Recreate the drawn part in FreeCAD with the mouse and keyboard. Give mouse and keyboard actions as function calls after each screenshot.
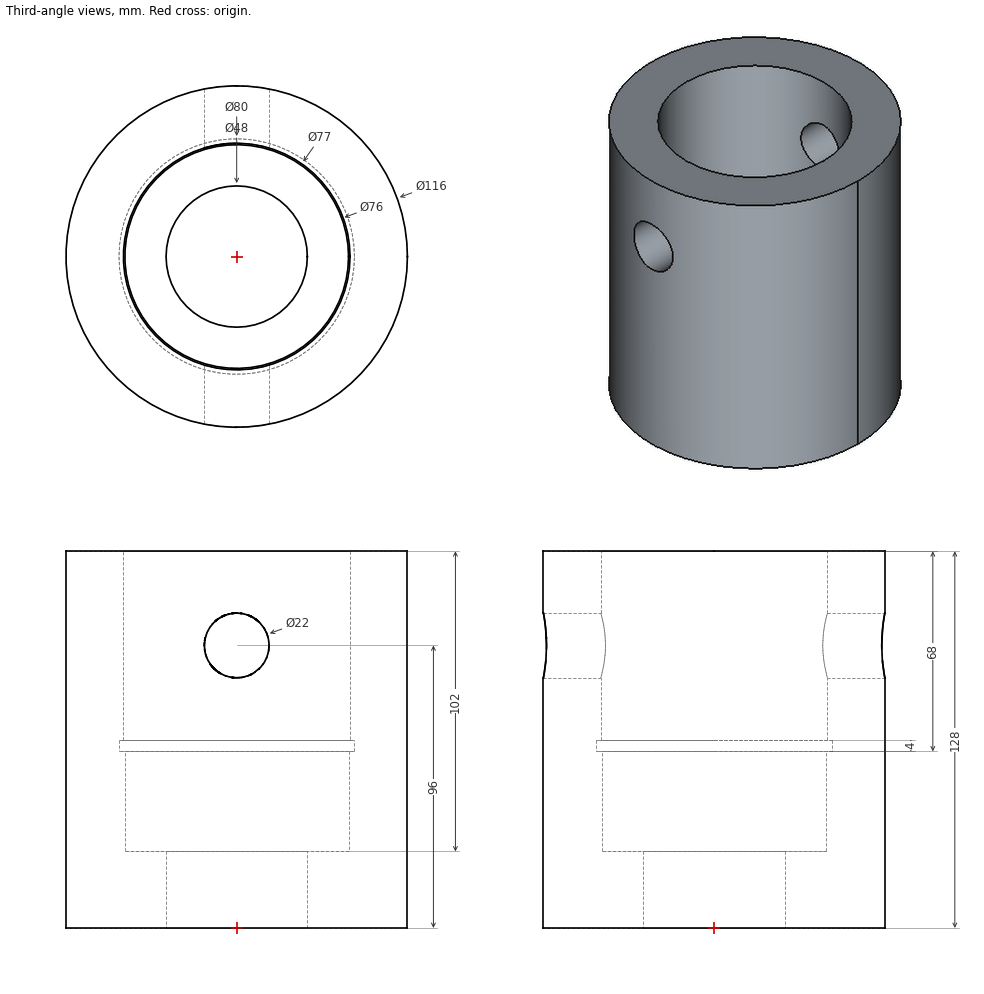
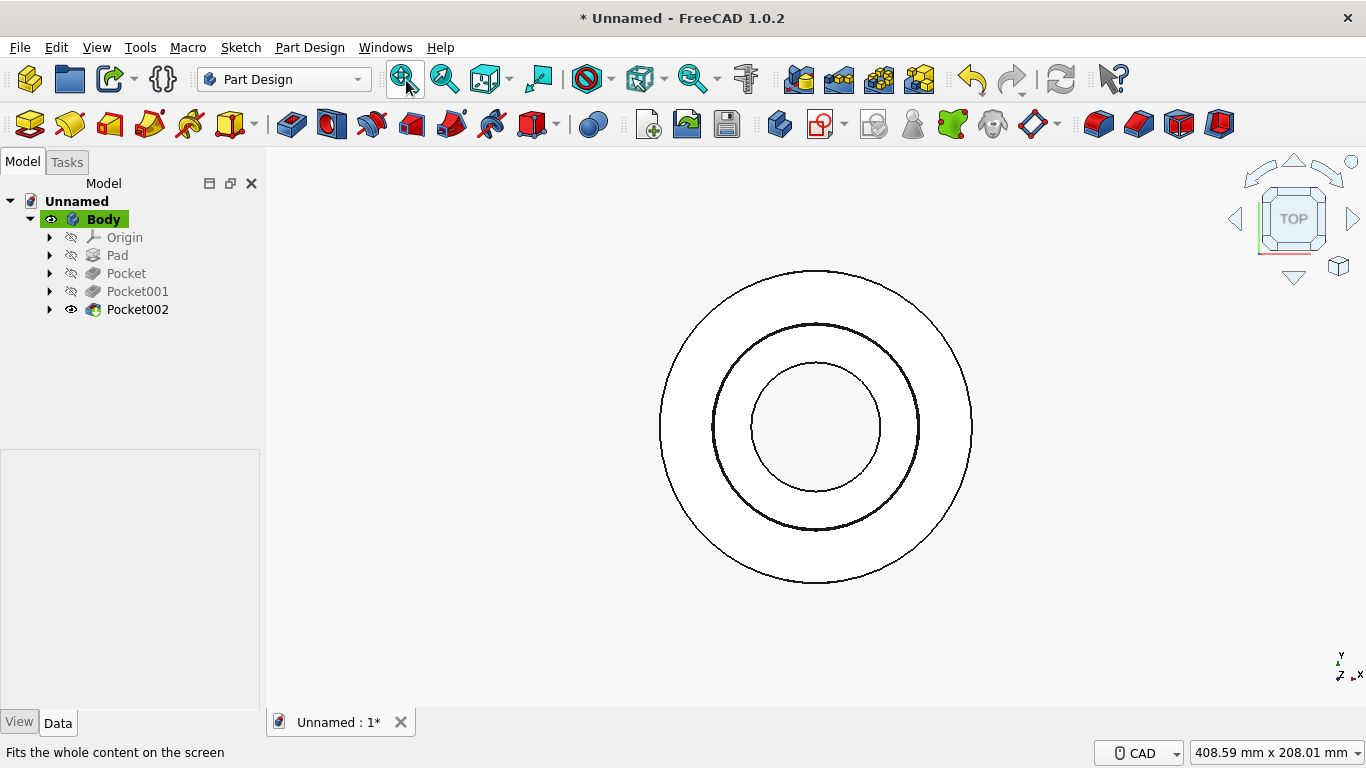
key(1)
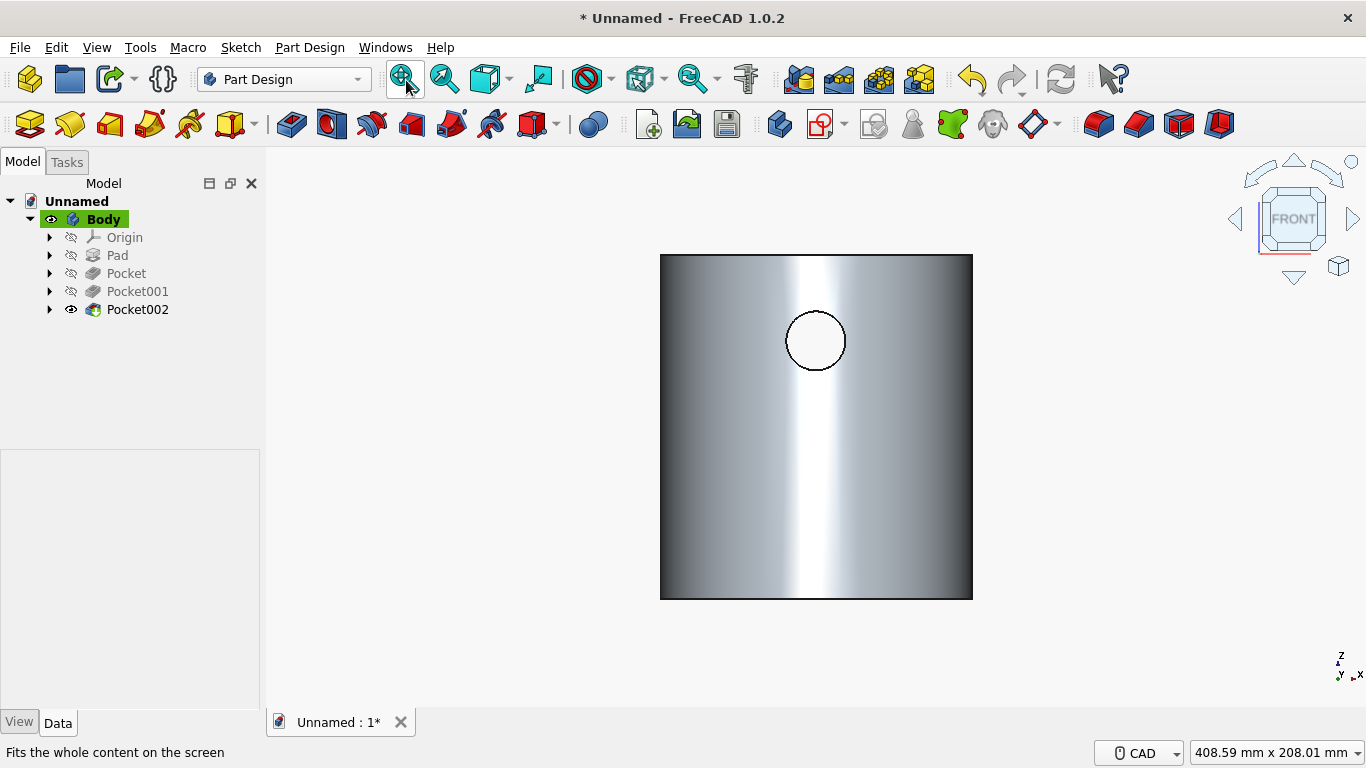
click(50, 237)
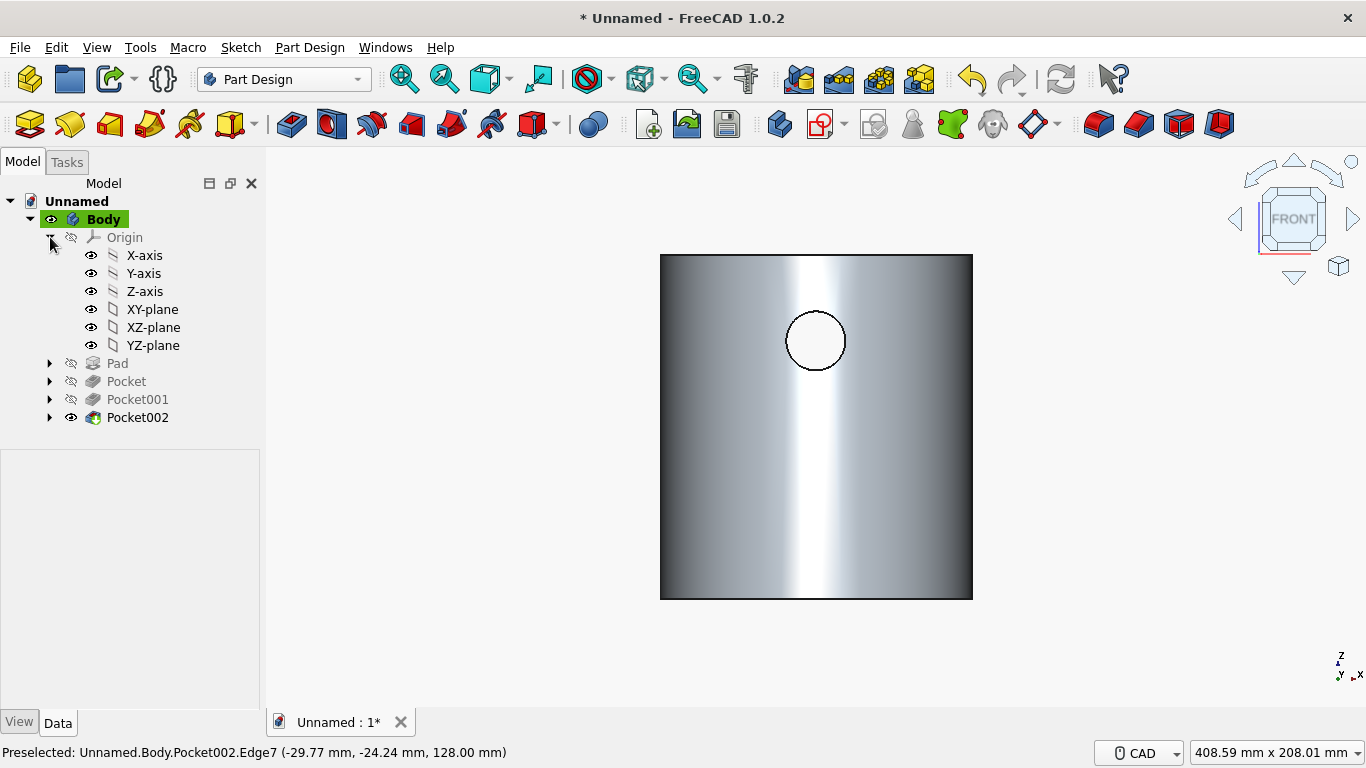
click(136, 309)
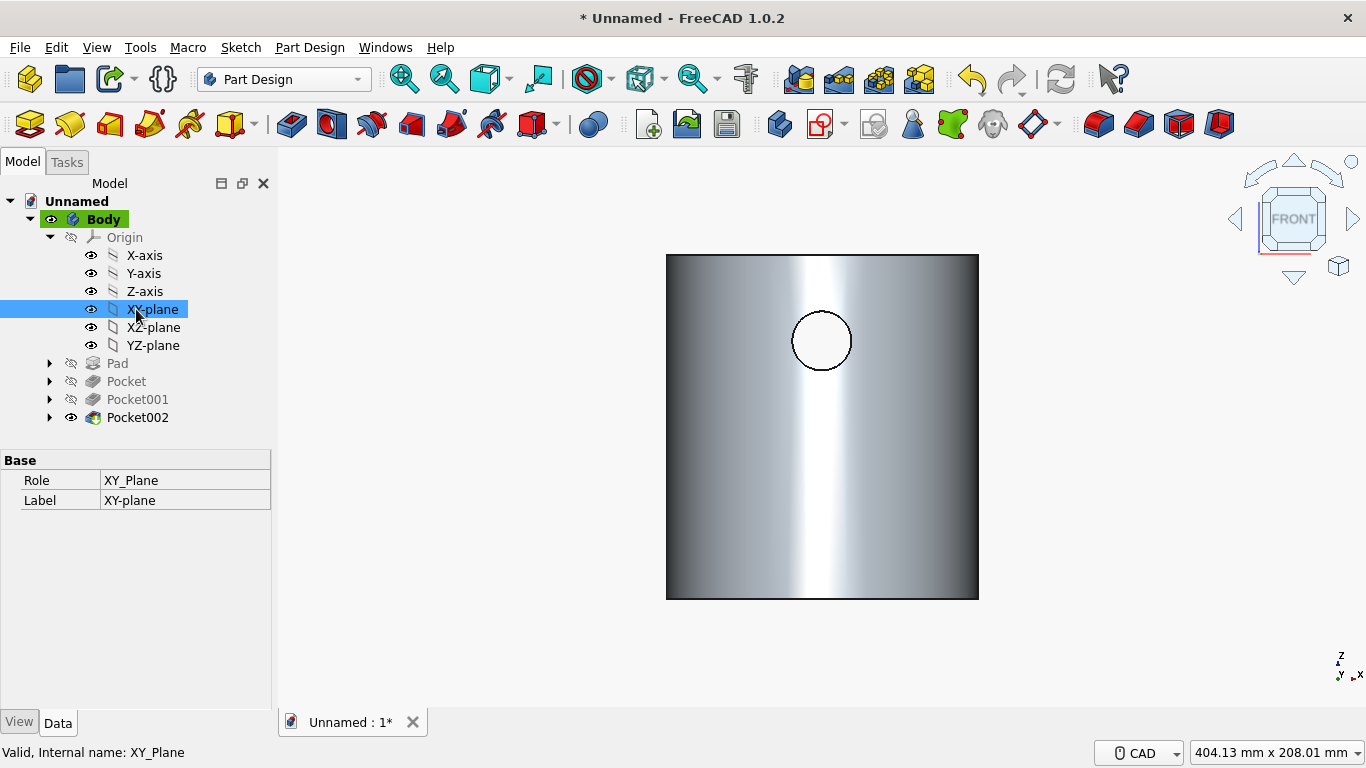
click(1034, 124)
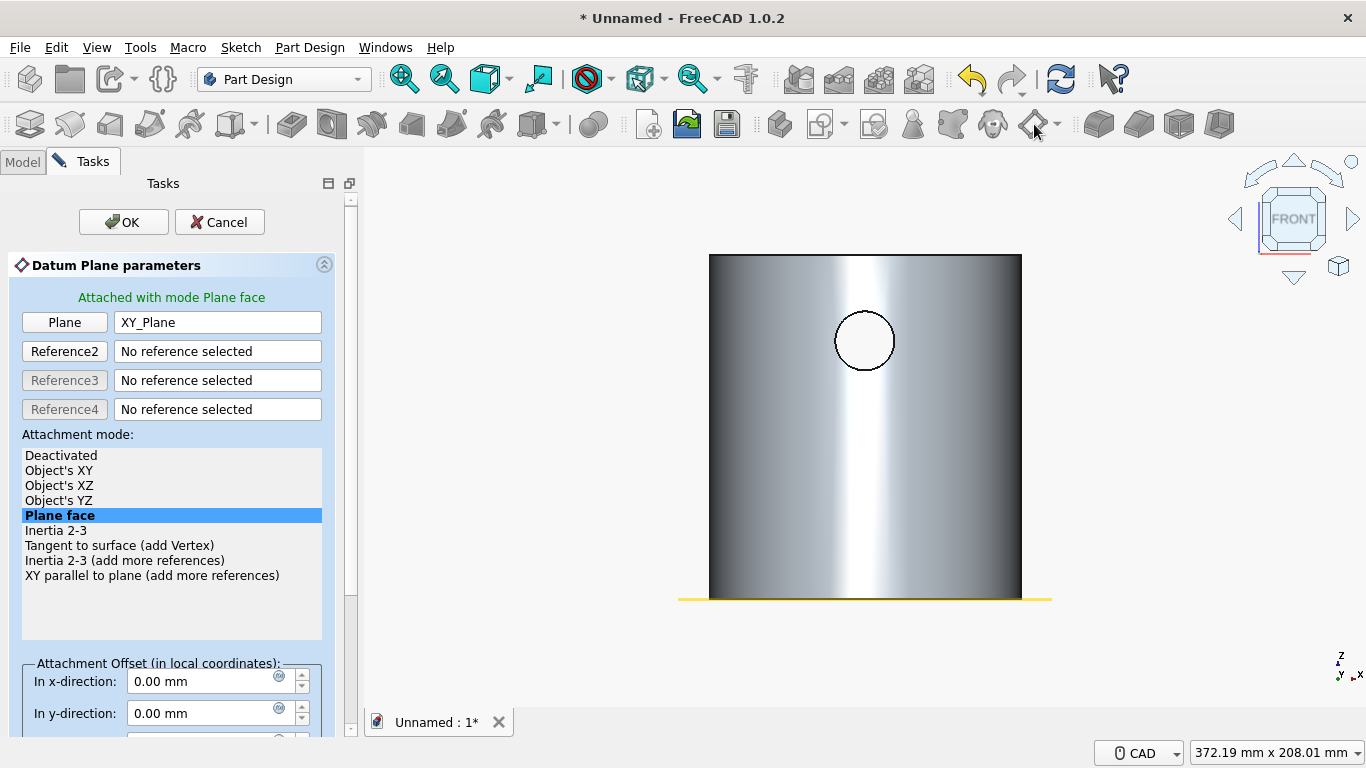
scroll(351, 464, down, 2)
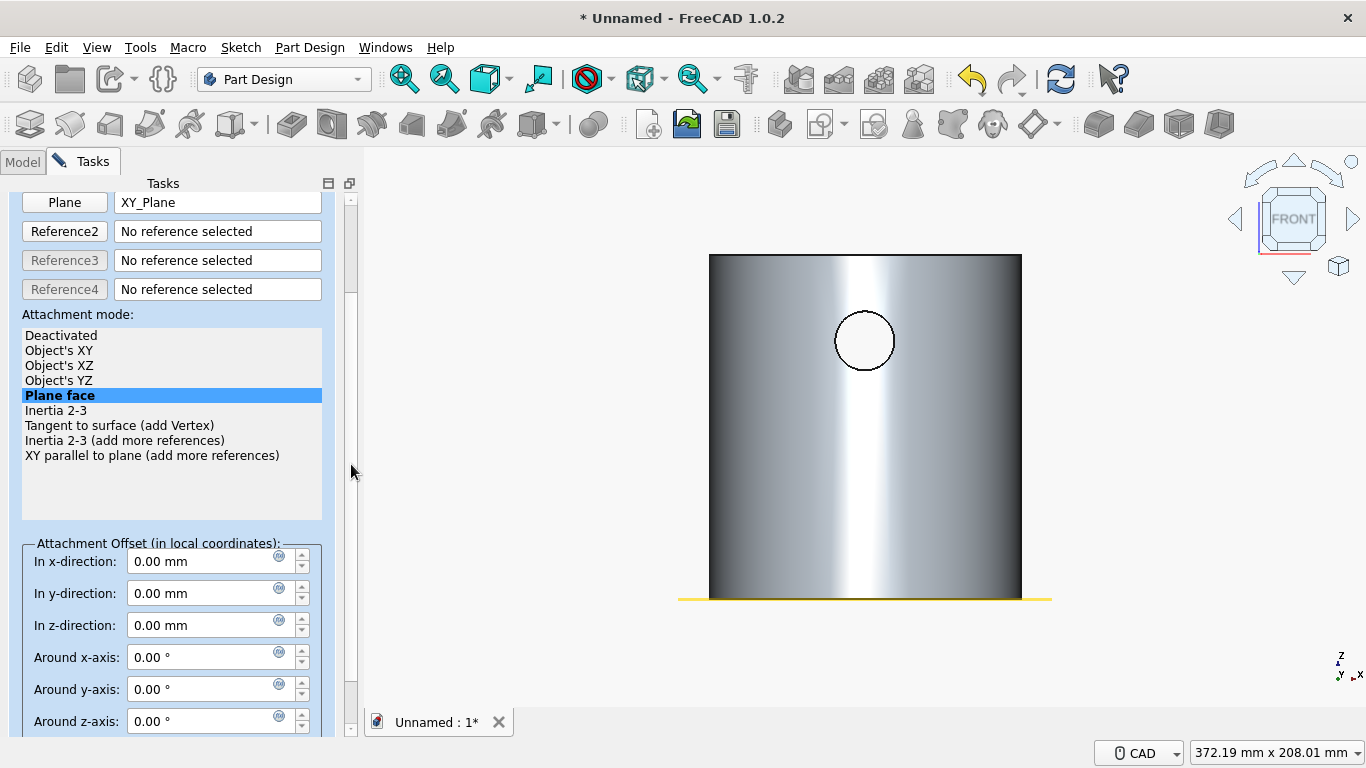
triple_click(210, 625)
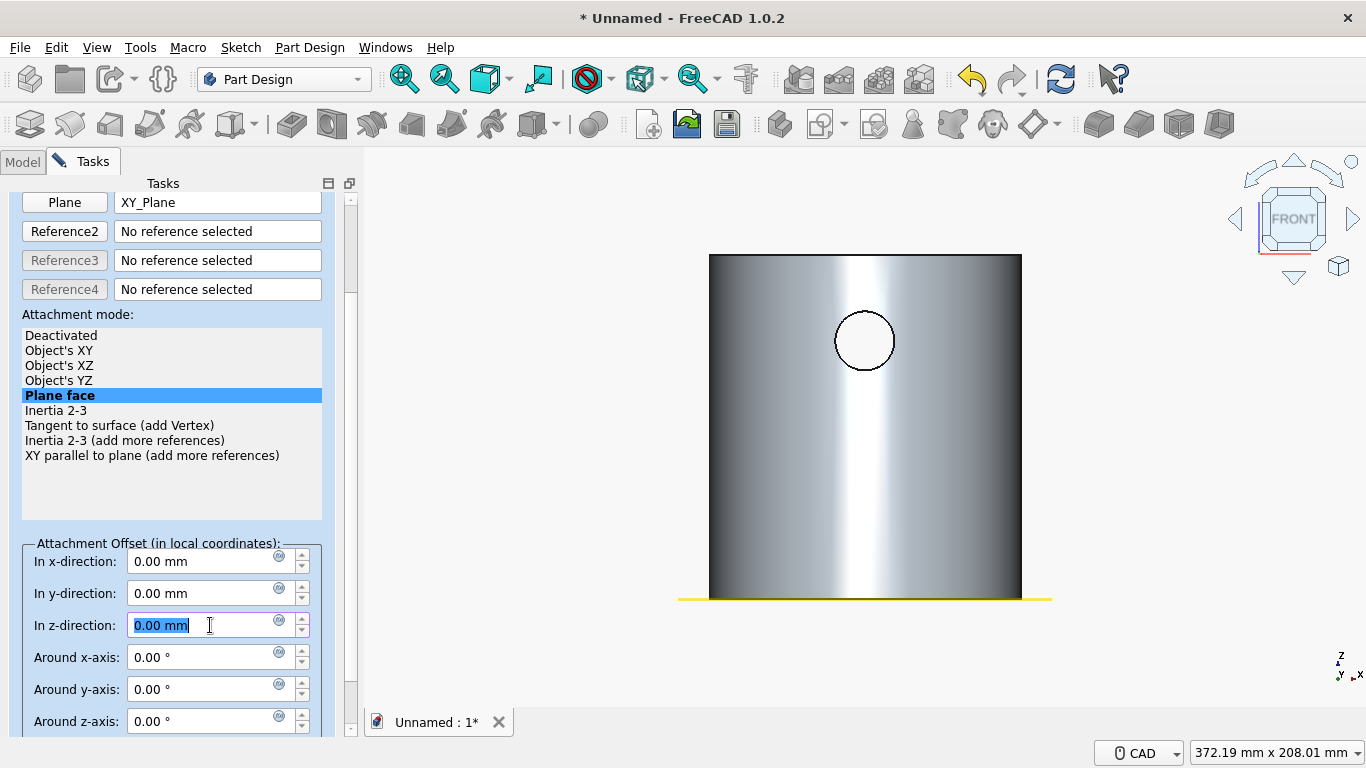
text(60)
key(Tab)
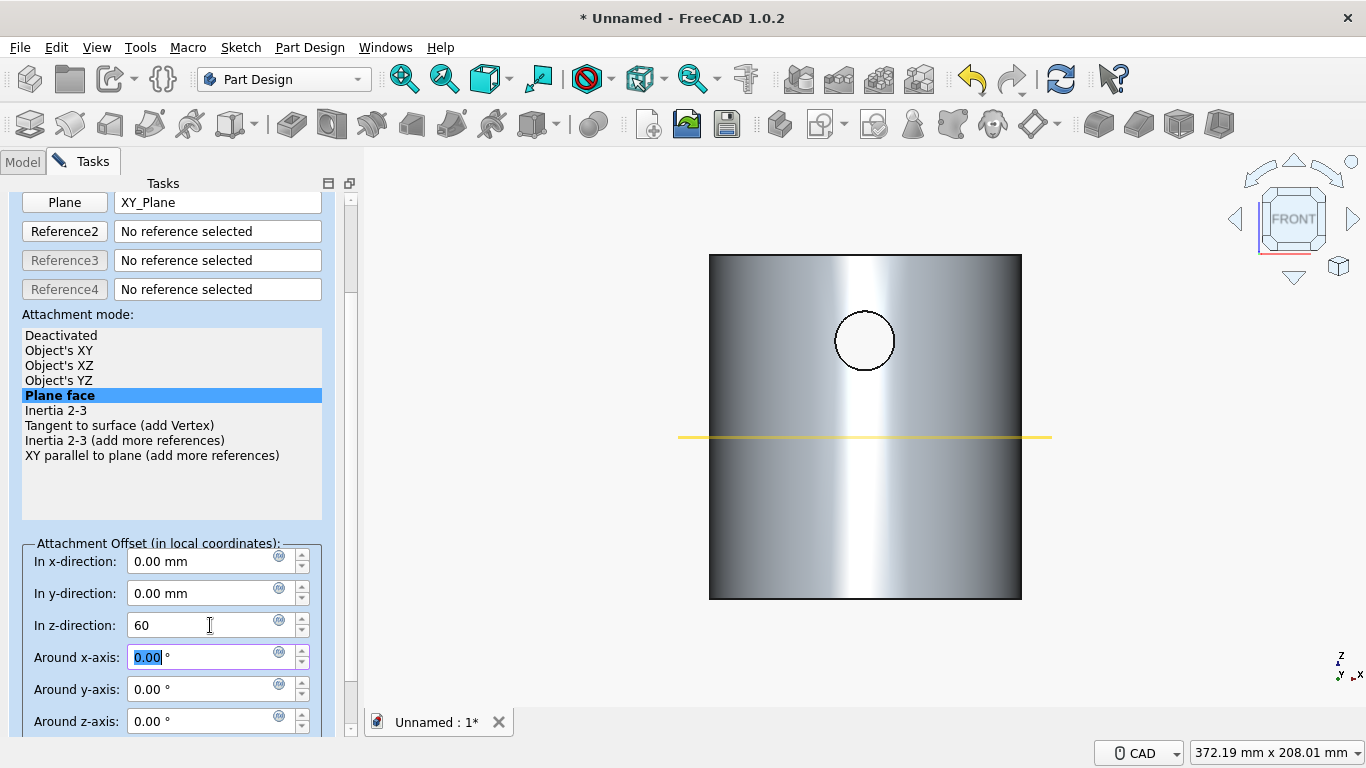
scroll(351, 464, up, 3)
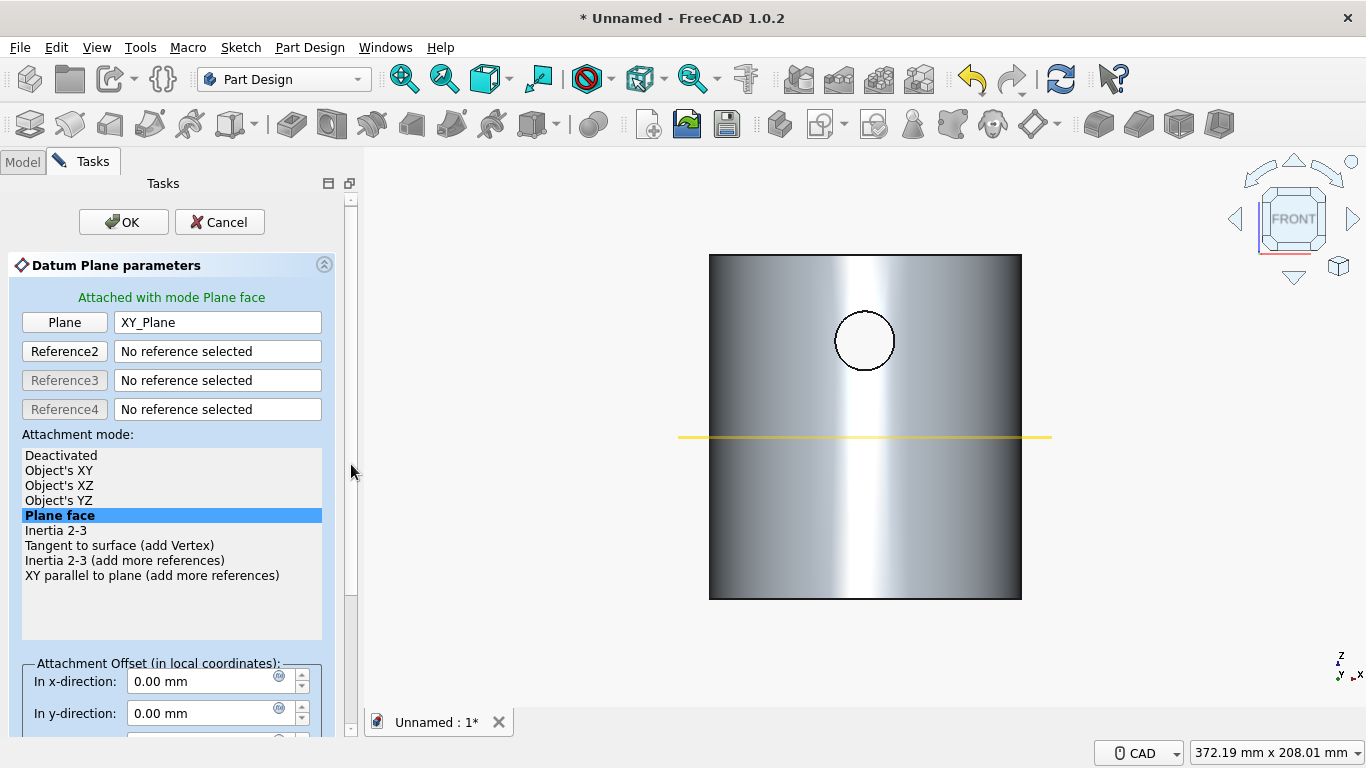
click(124, 222)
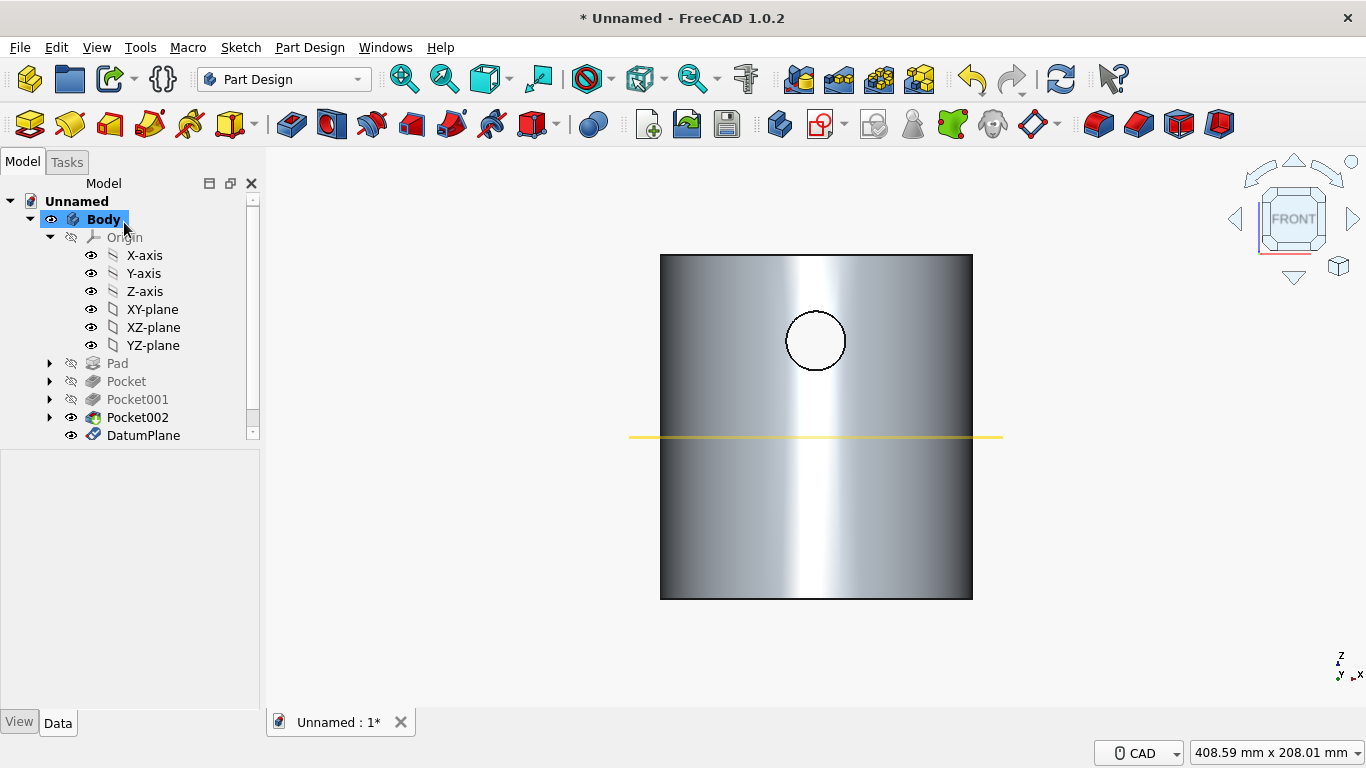
click(116, 435)